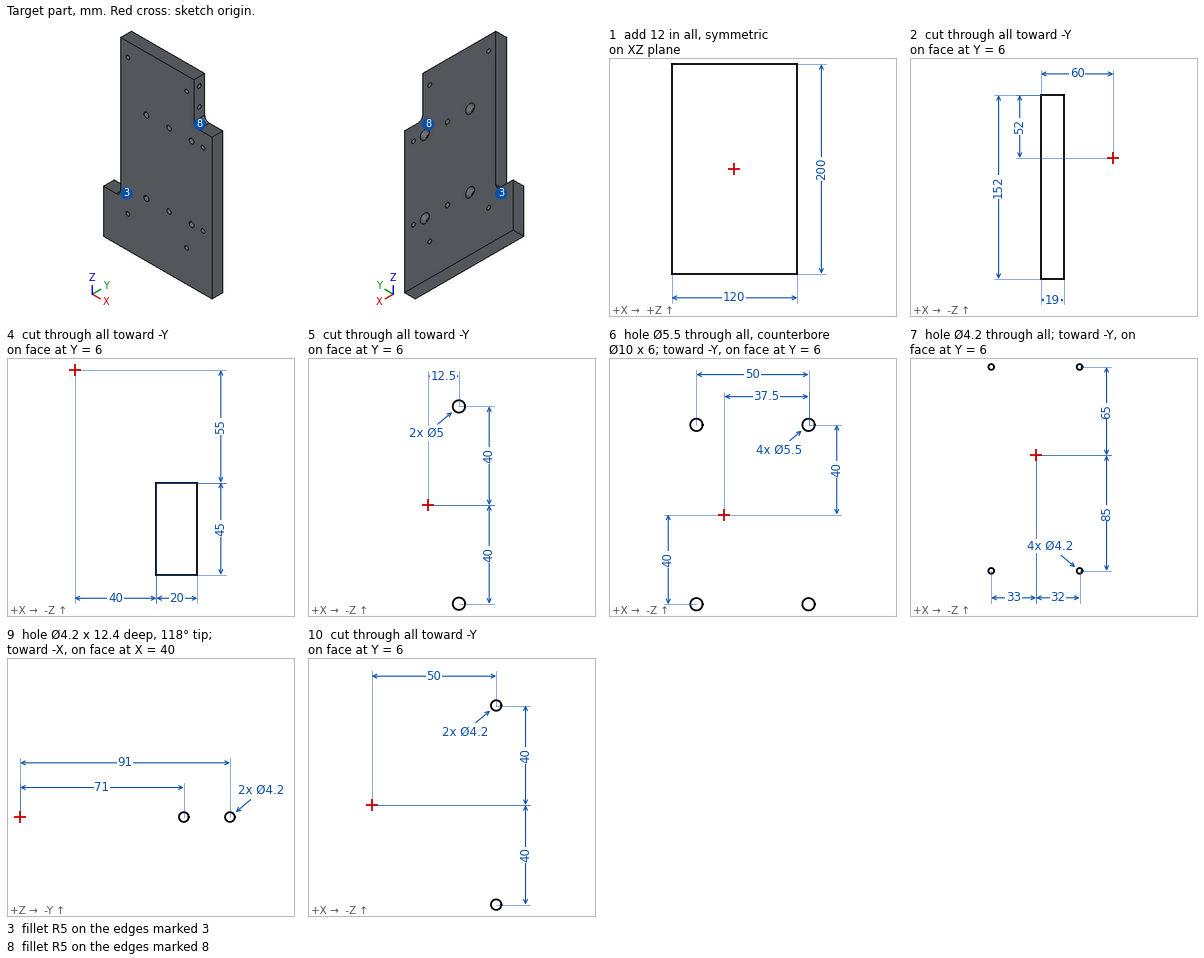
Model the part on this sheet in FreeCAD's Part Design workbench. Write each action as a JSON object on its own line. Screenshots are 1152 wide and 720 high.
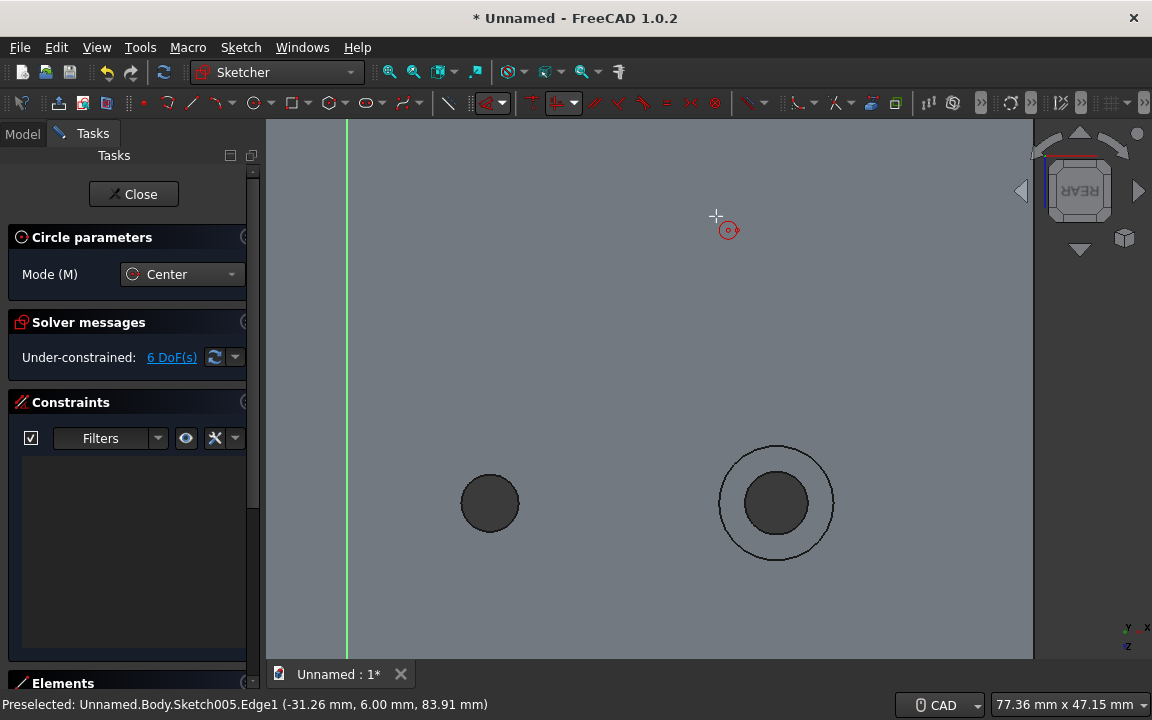
{"action": "scroll", "coordinate": [716, 215], "scroll_direction": "down", "scroll_amount": 8}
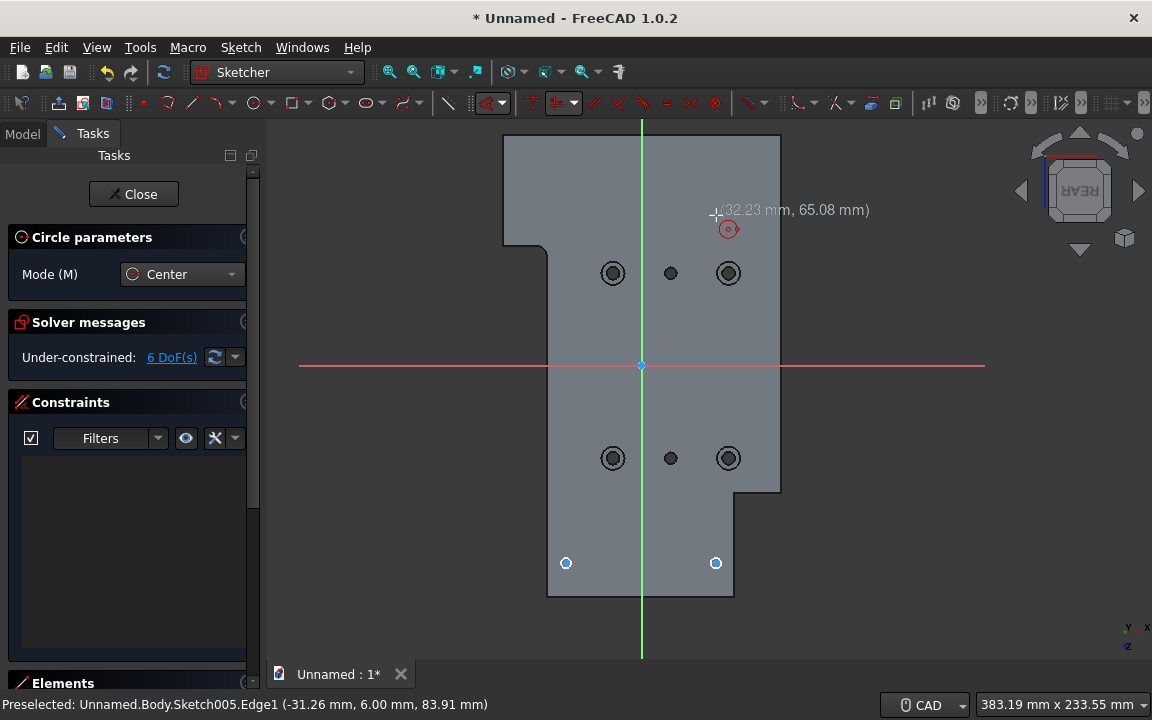
{"action": "left_click", "coordinate": [716, 216]}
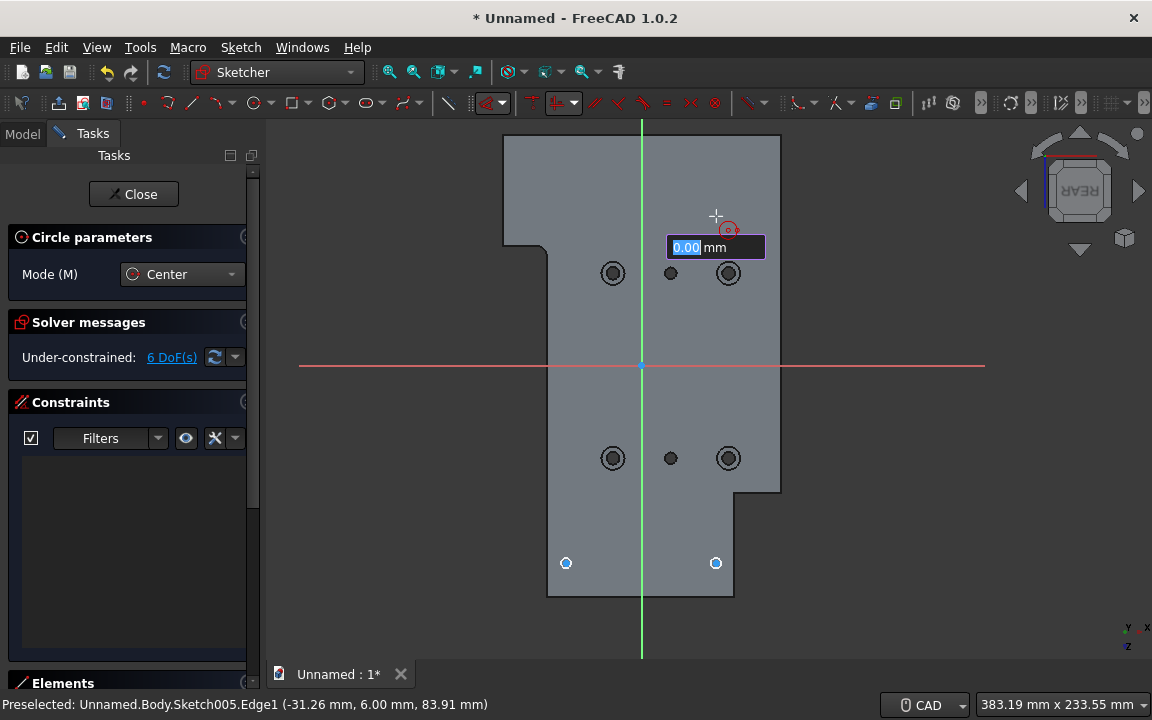
{"action": "scroll", "coordinate": [719, 212], "scroll_direction": "up", "scroll_amount": 6}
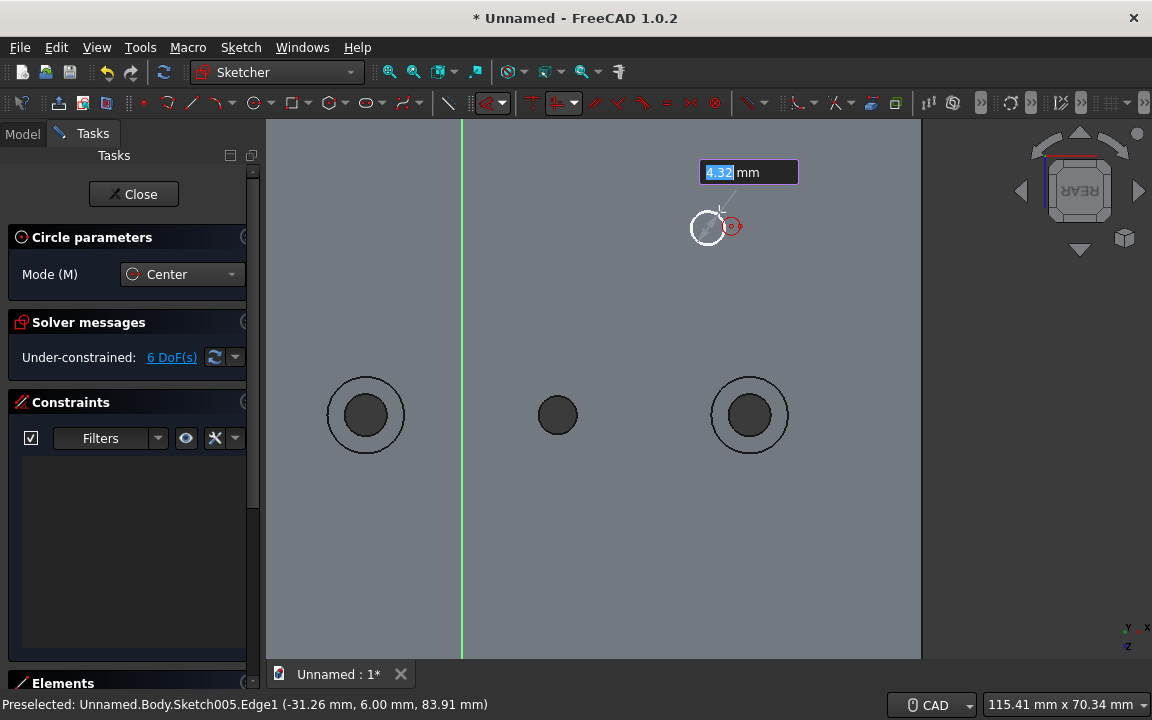
{"action": "left_click", "coordinate": [719, 212]}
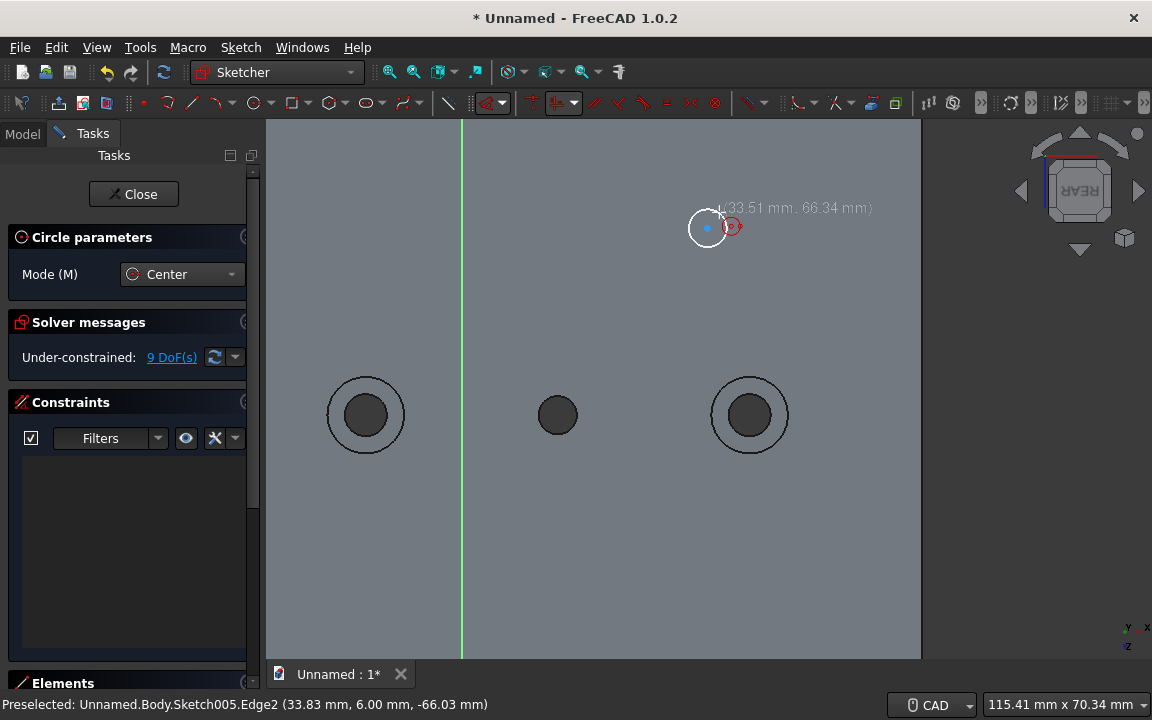
{"action": "scroll", "coordinate": [719, 212], "scroll_direction": "down", "scroll_amount": 6}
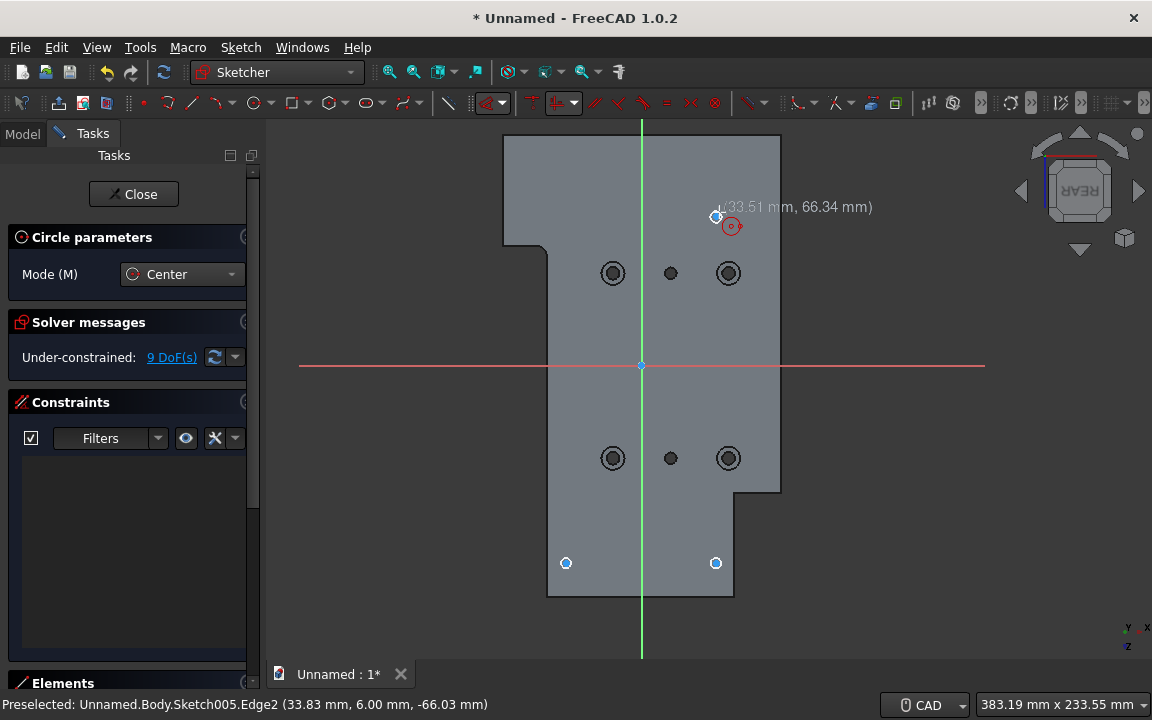
{"action": "scroll", "coordinate": [566, 216], "scroll_direction": "up", "scroll_amount": 8}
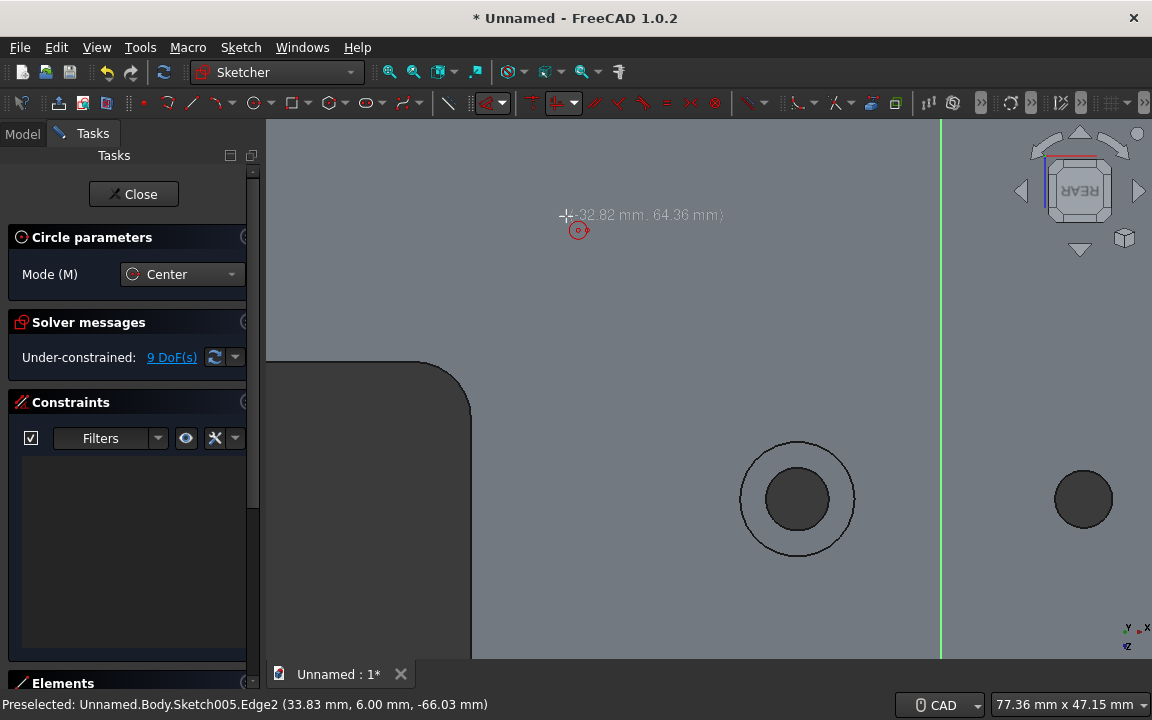
{"action": "scroll", "coordinate": [566, 216], "scroll_direction": "down", "scroll_amount": 8}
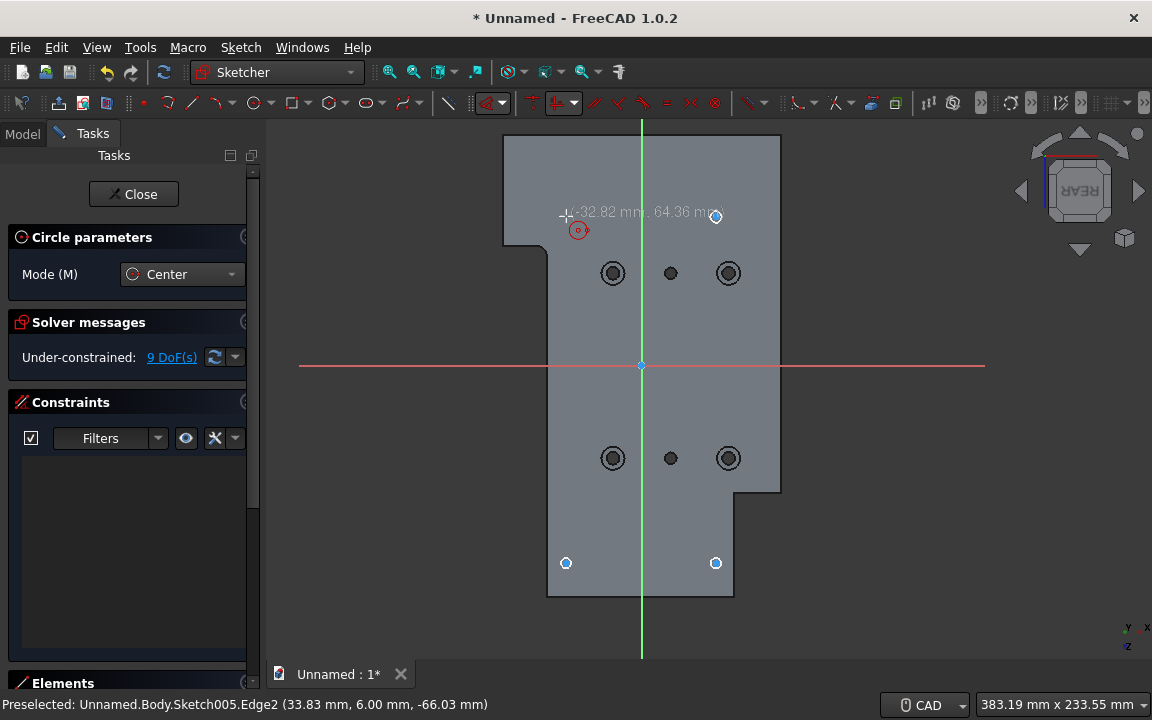
{"action": "left_click", "coordinate": [566, 216]}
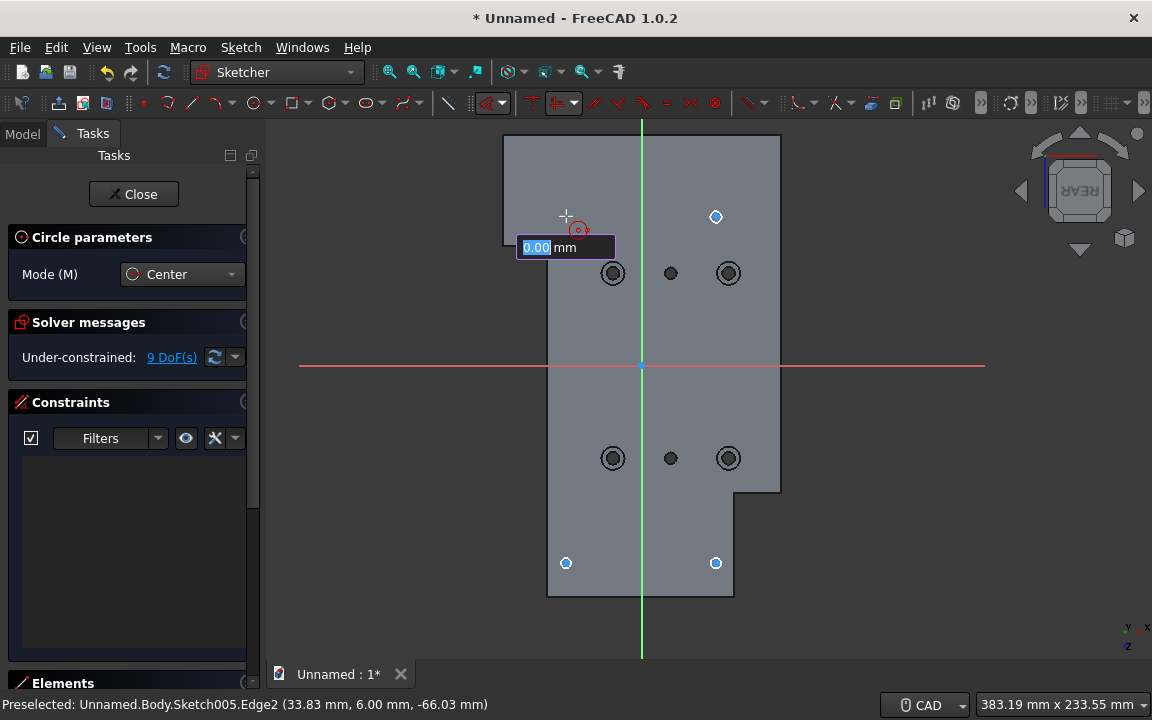
{"action": "scroll", "coordinate": [569, 212], "scroll_direction": "up", "scroll_amount": 6}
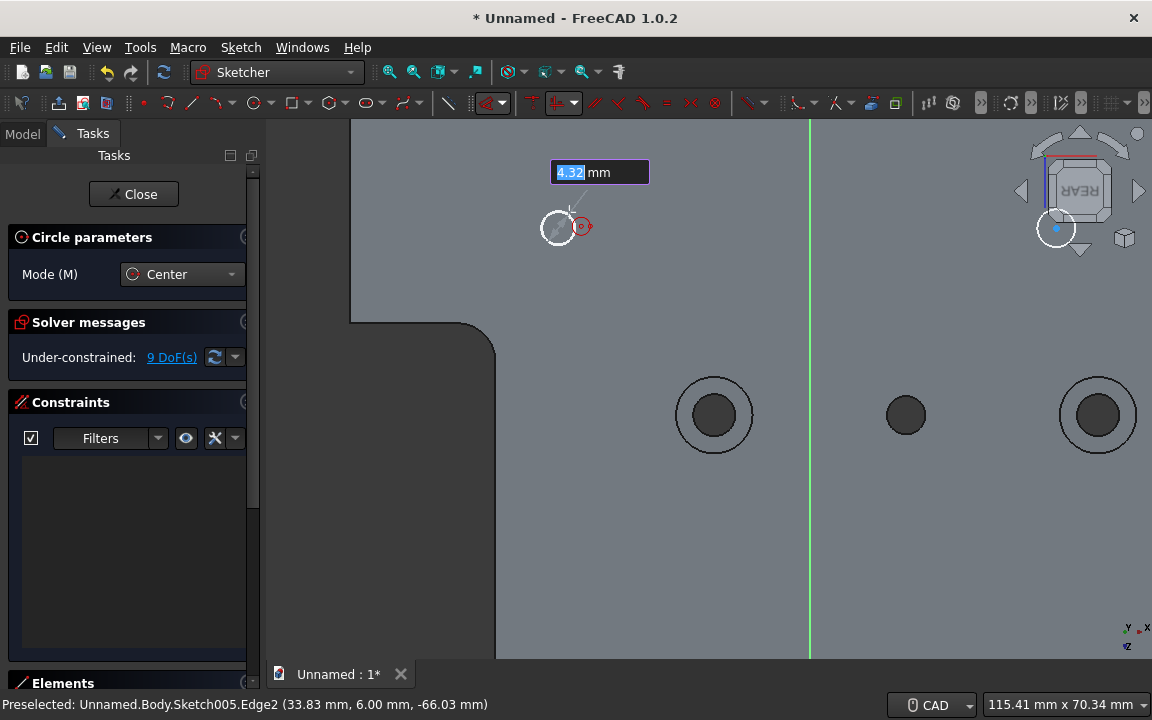
{"action": "left_click", "coordinate": [568, 212]}
{"action": "key", "text": "Escape"}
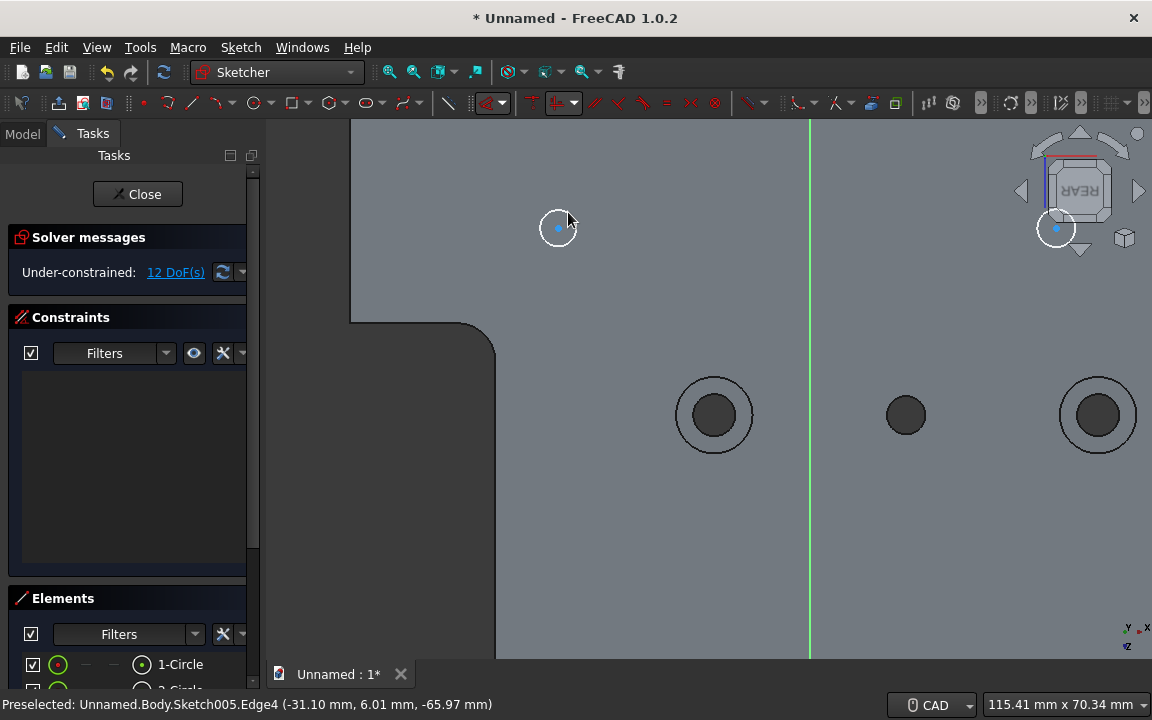
{"action": "scroll", "coordinate": [569, 212], "scroll_direction": "down", "scroll_amount": 6}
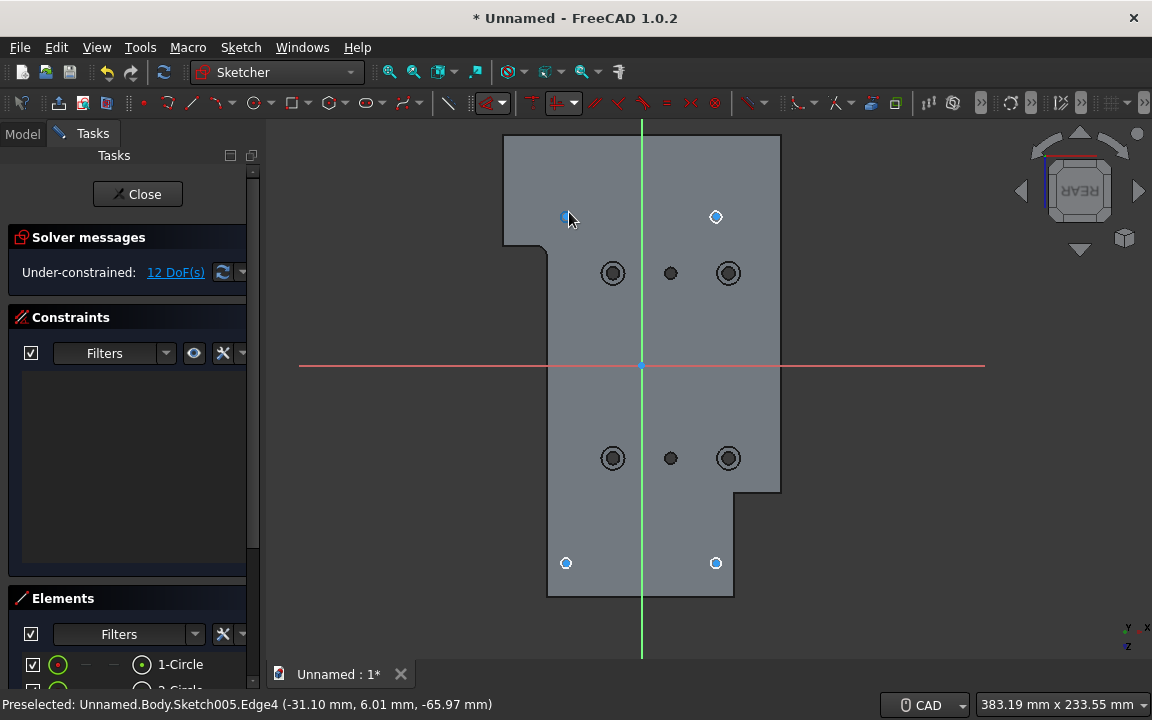
{"action": "scroll", "coordinate": [720, 559], "scroll_direction": "up", "scroll_amount": 5}